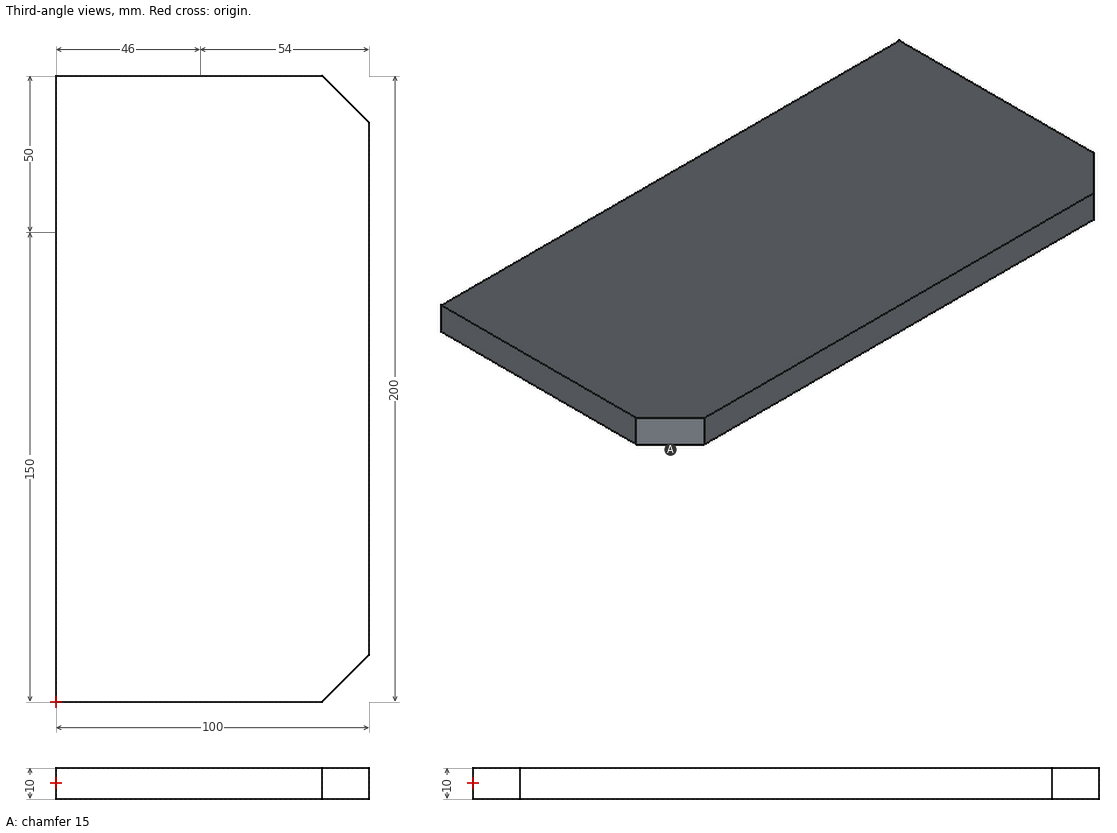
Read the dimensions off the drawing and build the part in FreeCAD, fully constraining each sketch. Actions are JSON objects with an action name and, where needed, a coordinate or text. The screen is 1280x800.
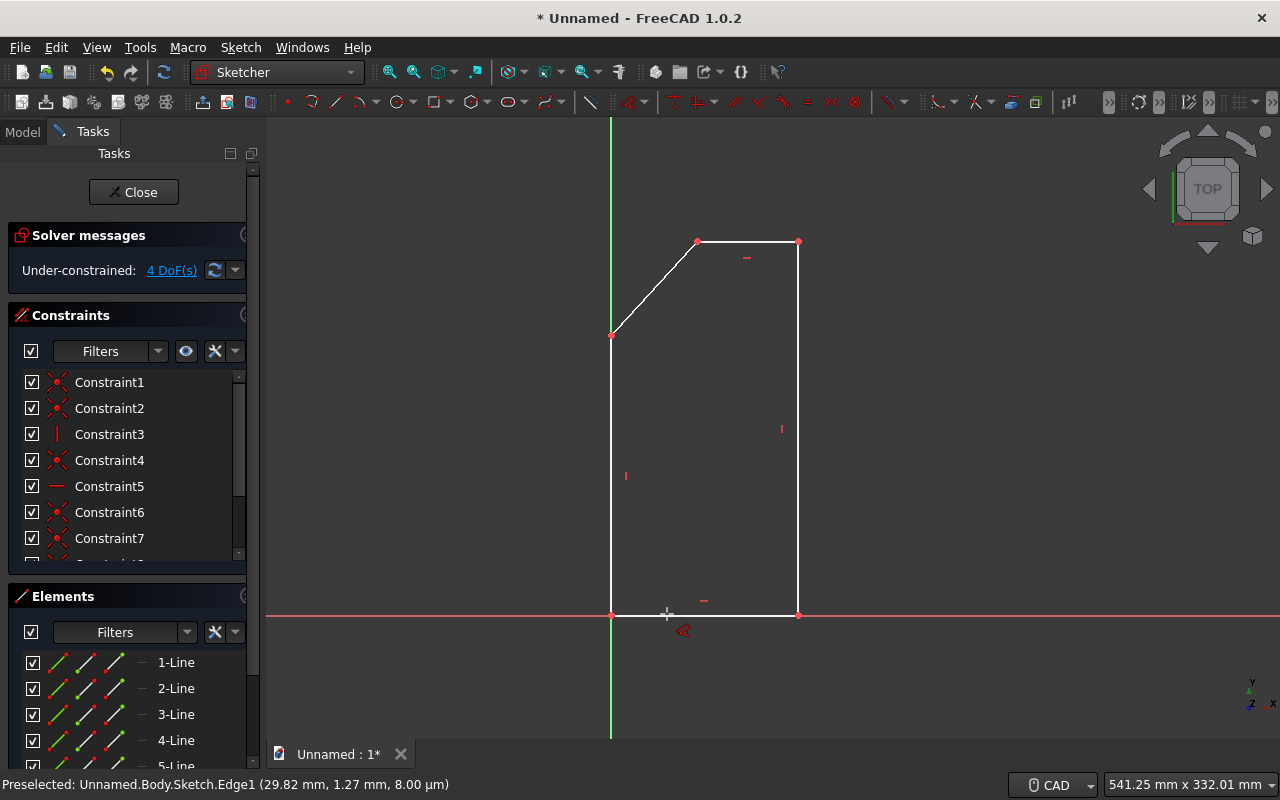
{"action": "left_click", "coordinate": [768, 242]}
{"action": "left_click", "coordinate": [747, 208]}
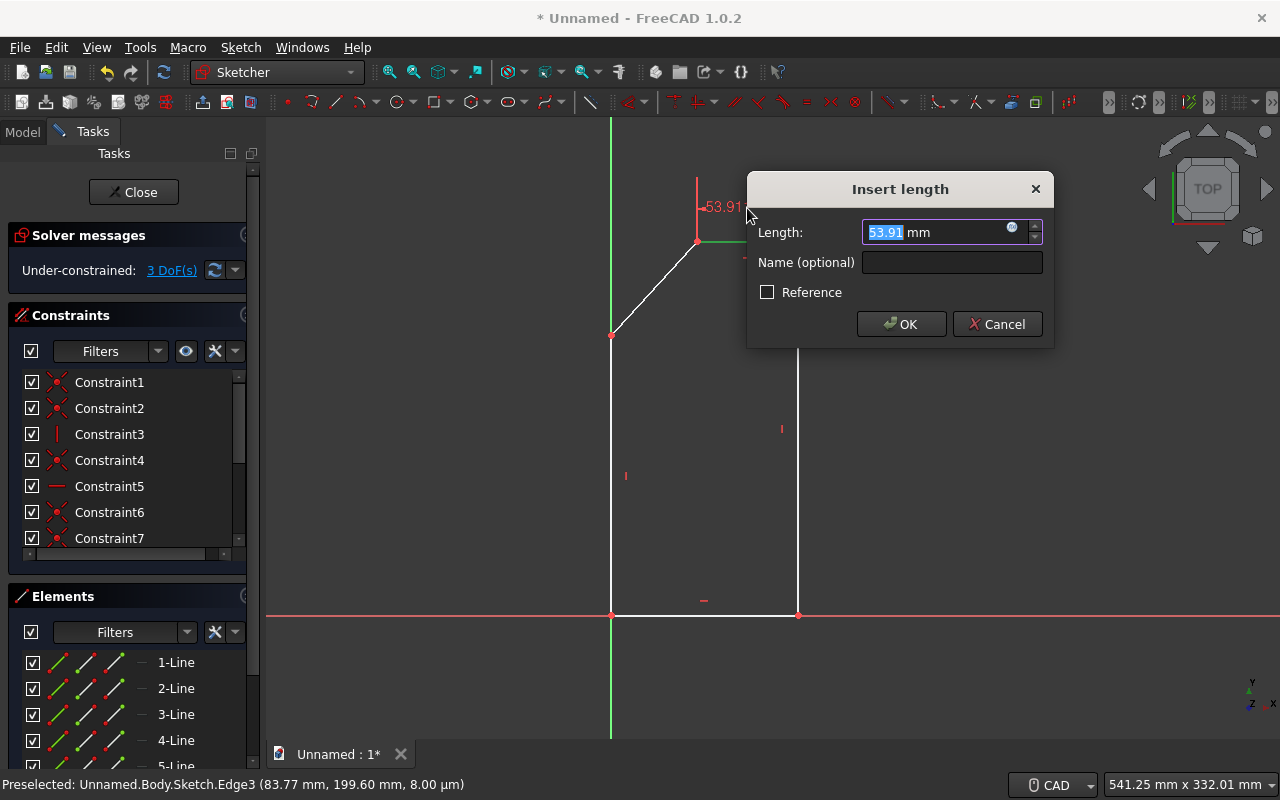
{"action": "type", "text": "54"}
{"action": "key", "text": "Return"}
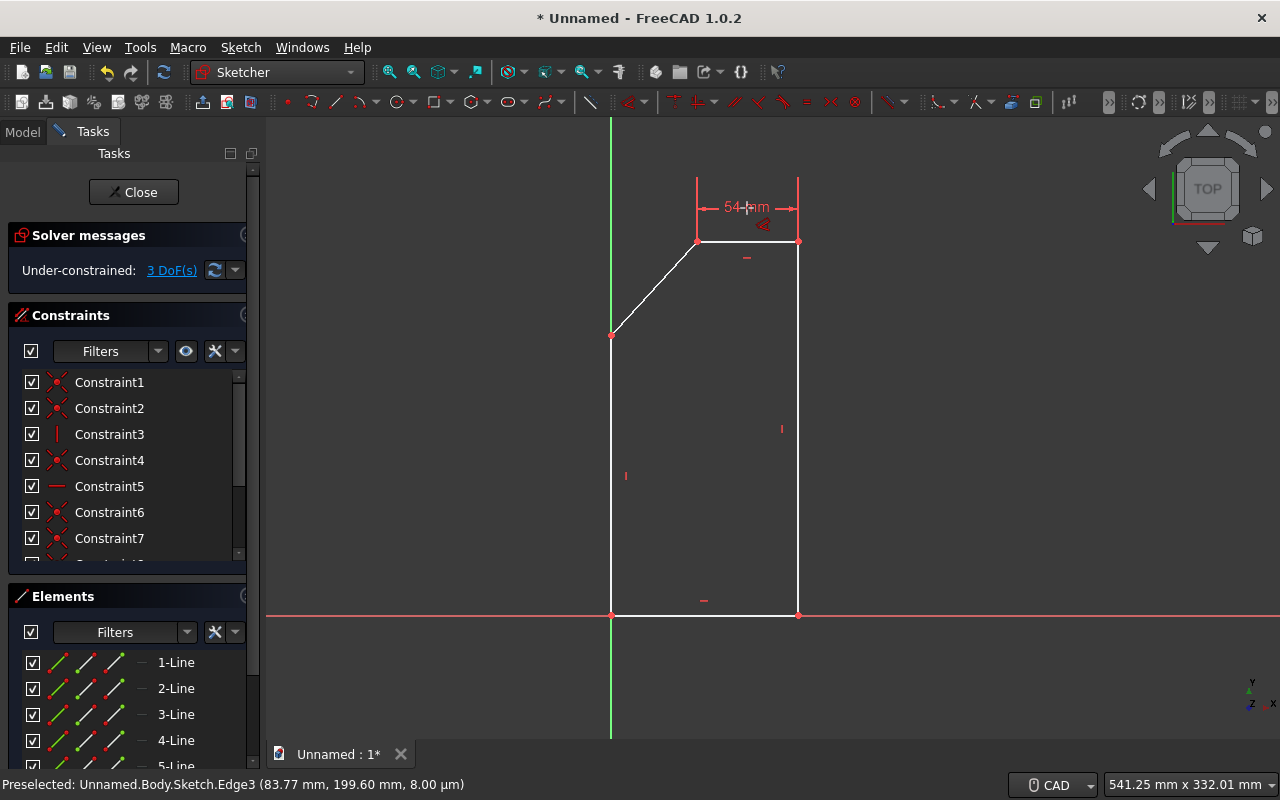
{"action": "left_click", "coordinate": [667, 616]}
{"action": "left_click", "coordinate": [705, 650]}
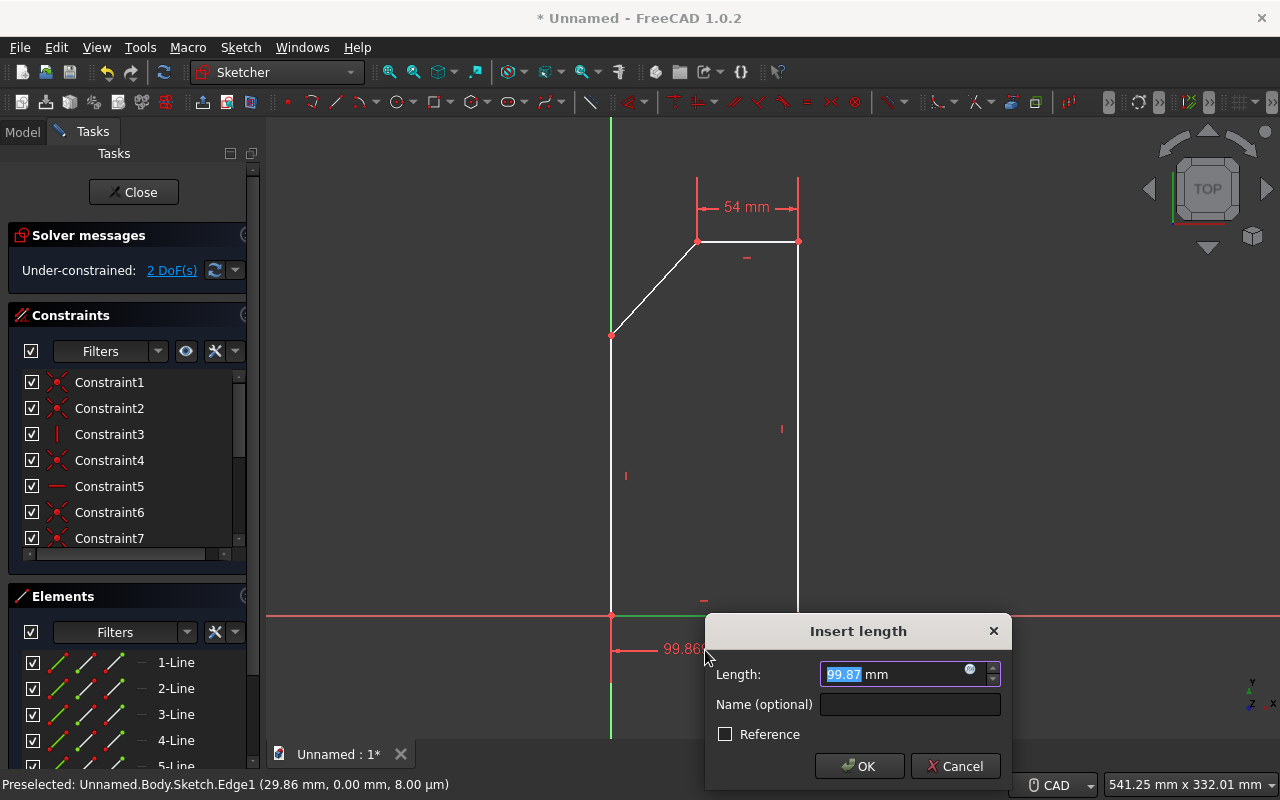
{"action": "type", "text": "100"}
{"action": "key", "text": "Return"}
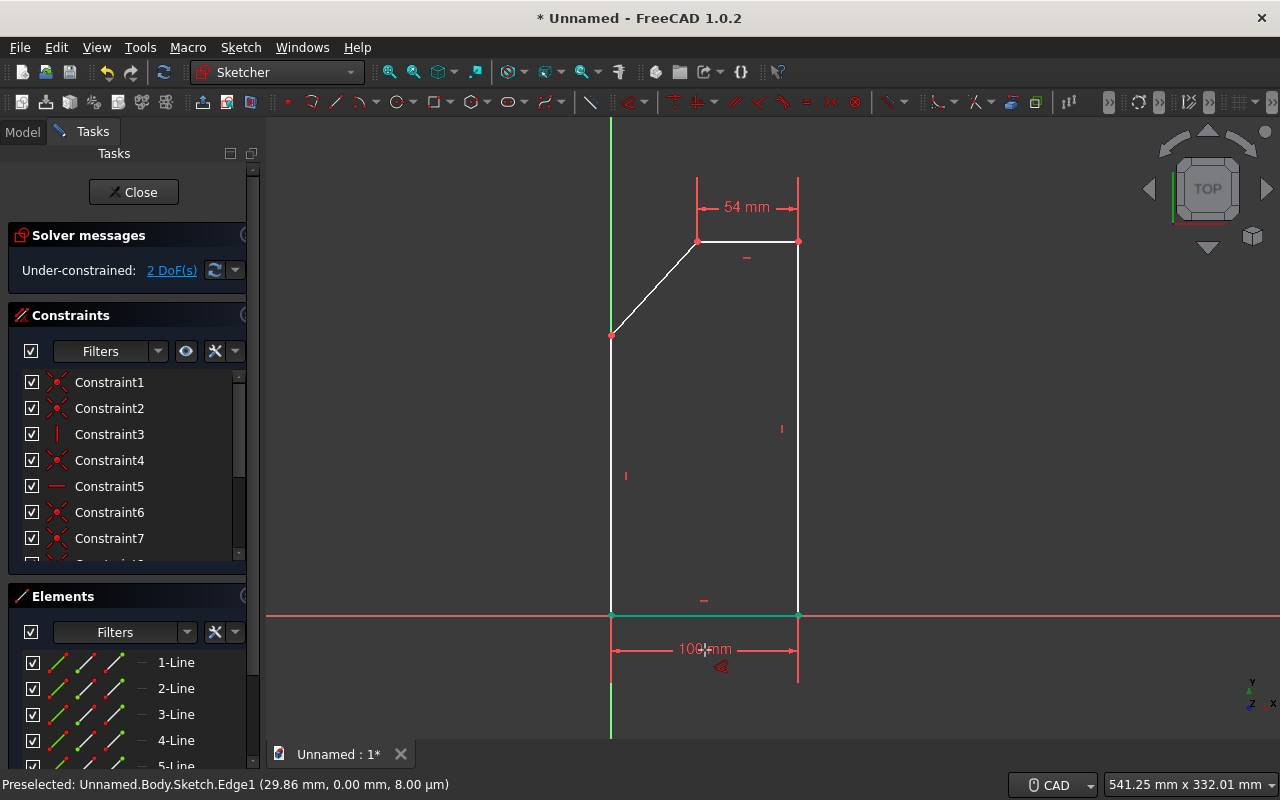
{"action": "left_click", "coordinate": [798, 504]}
{"action": "left_click", "coordinate": [832, 429]}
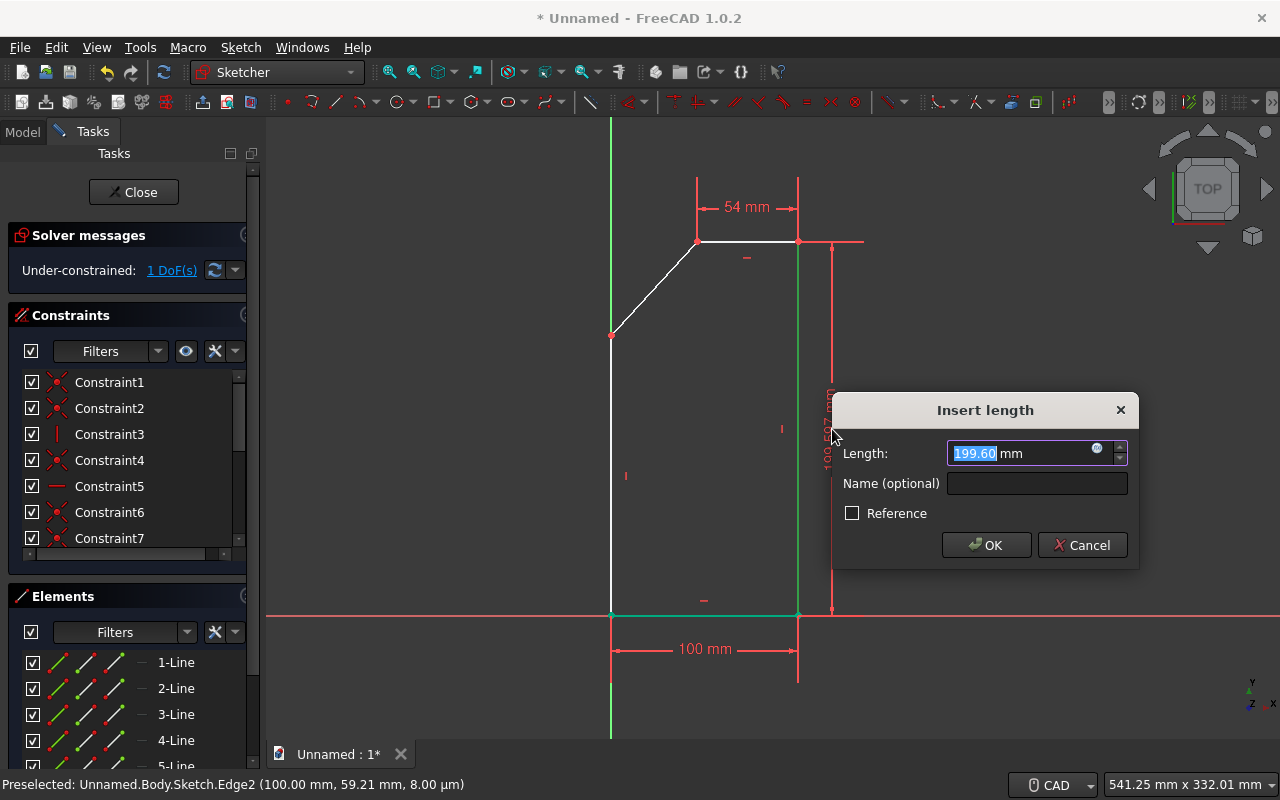
{"action": "type", "text": "200"}
{"action": "key", "text": "Return"}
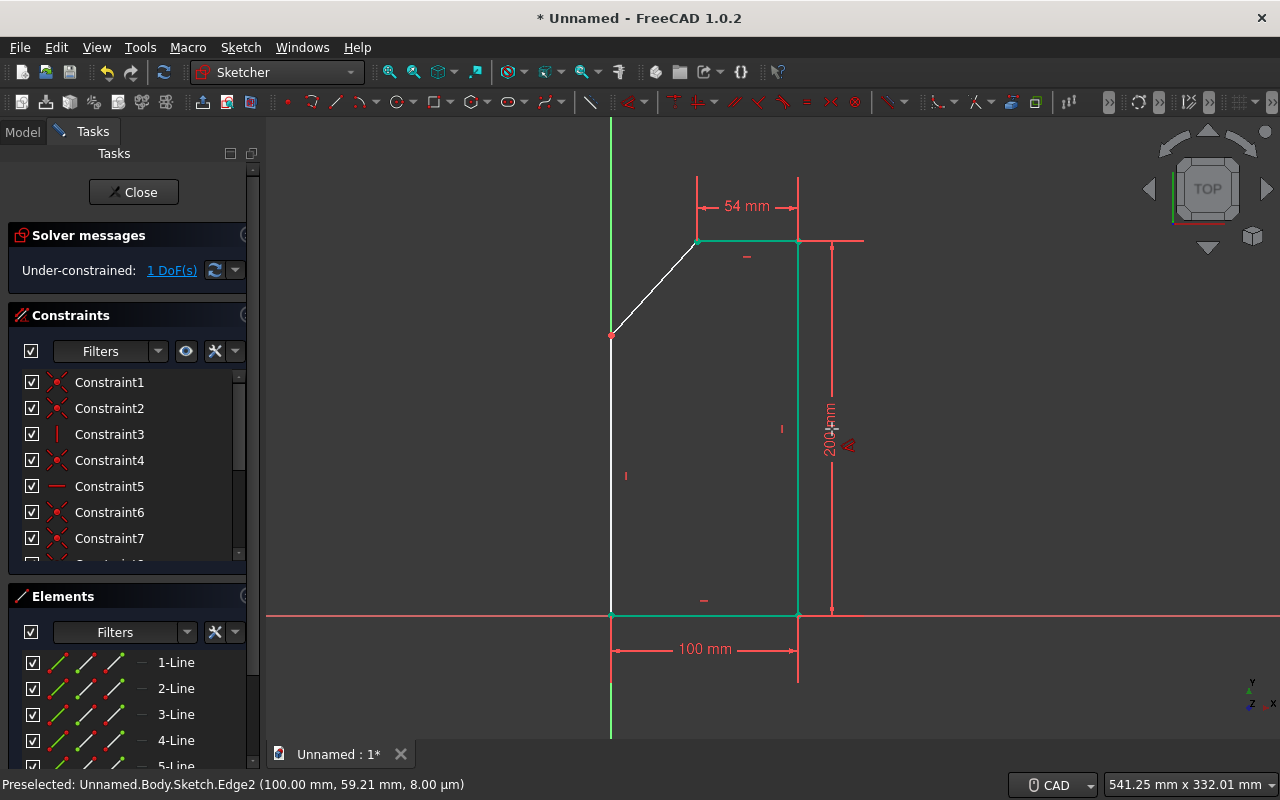
{"action": "left_click", "coordinate": [611, 420]}
{"action": "left_click", "coordinate": [577, 476]}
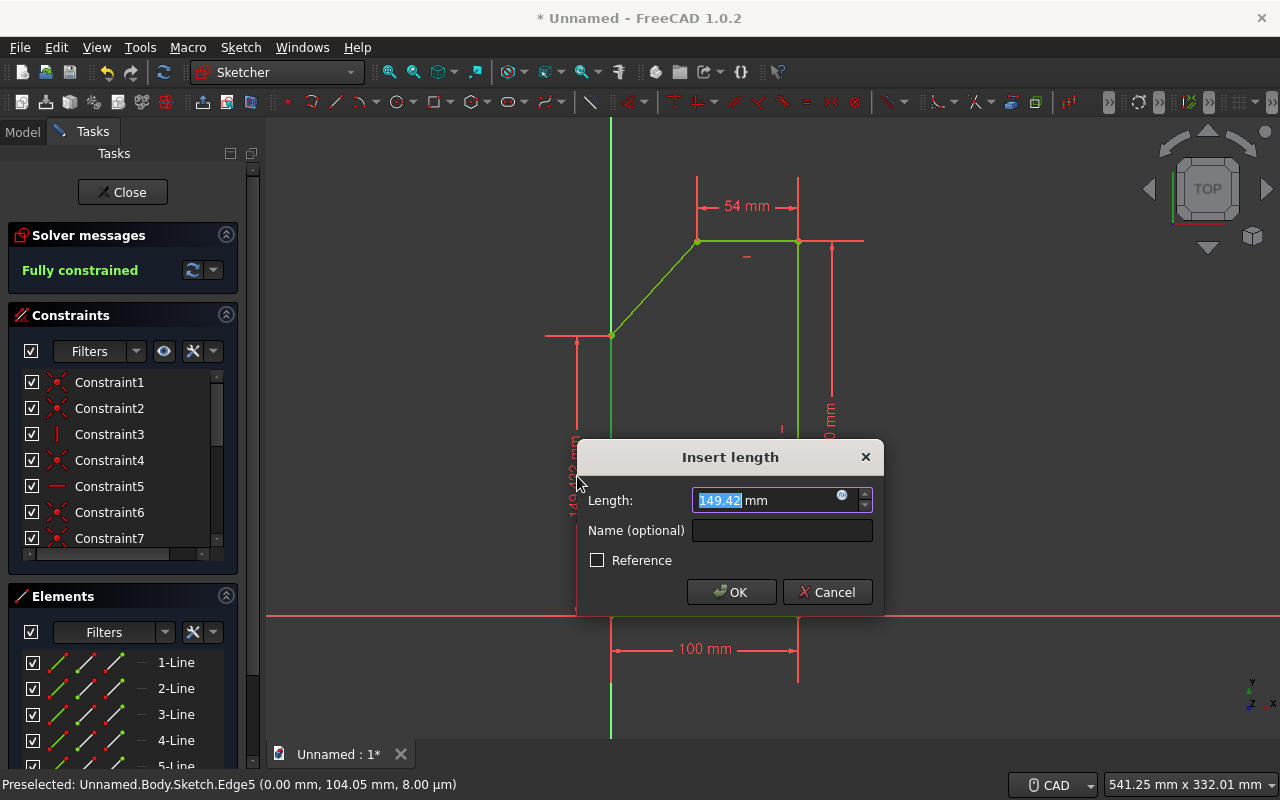
{"action": "type", "text": "150"}
{"action": "key", "text": "Return"}
{"action": "key", "text": "Escape"}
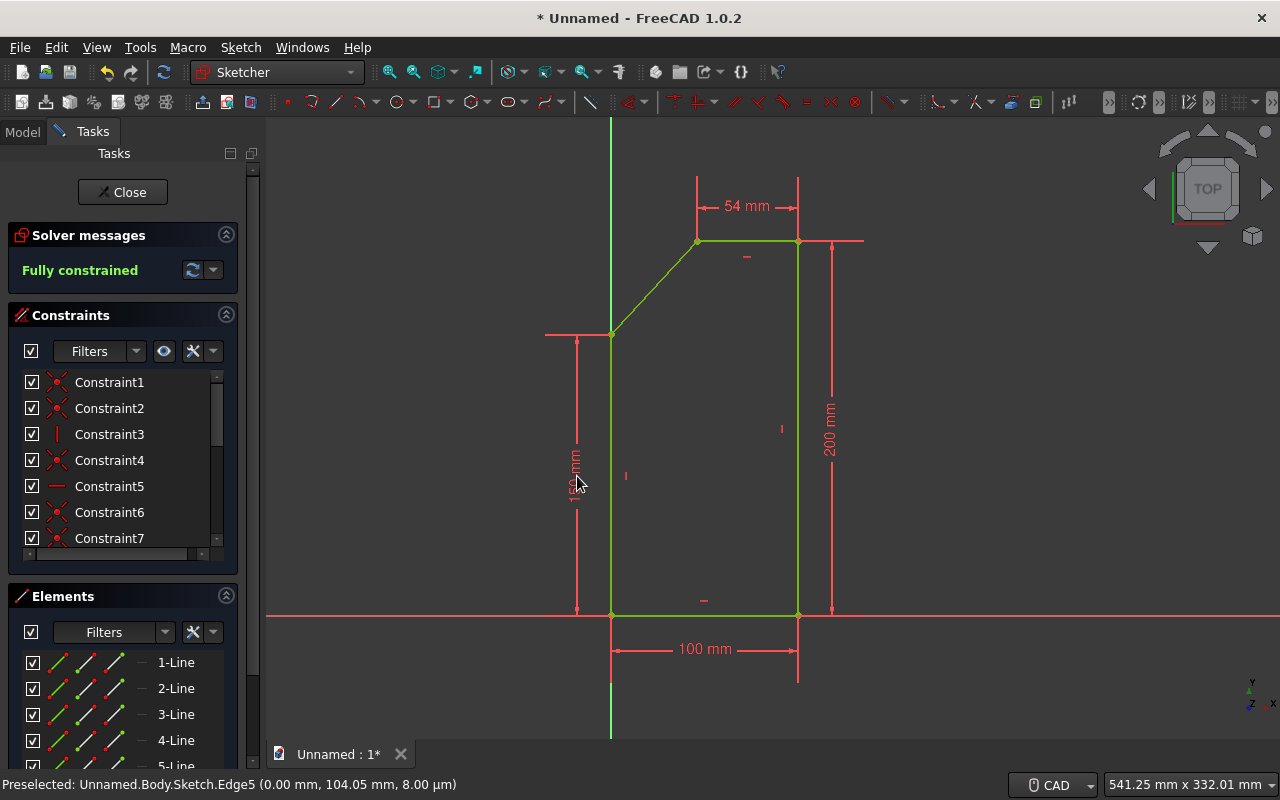
{"action": "left_click", "coordinate": [123, 192]}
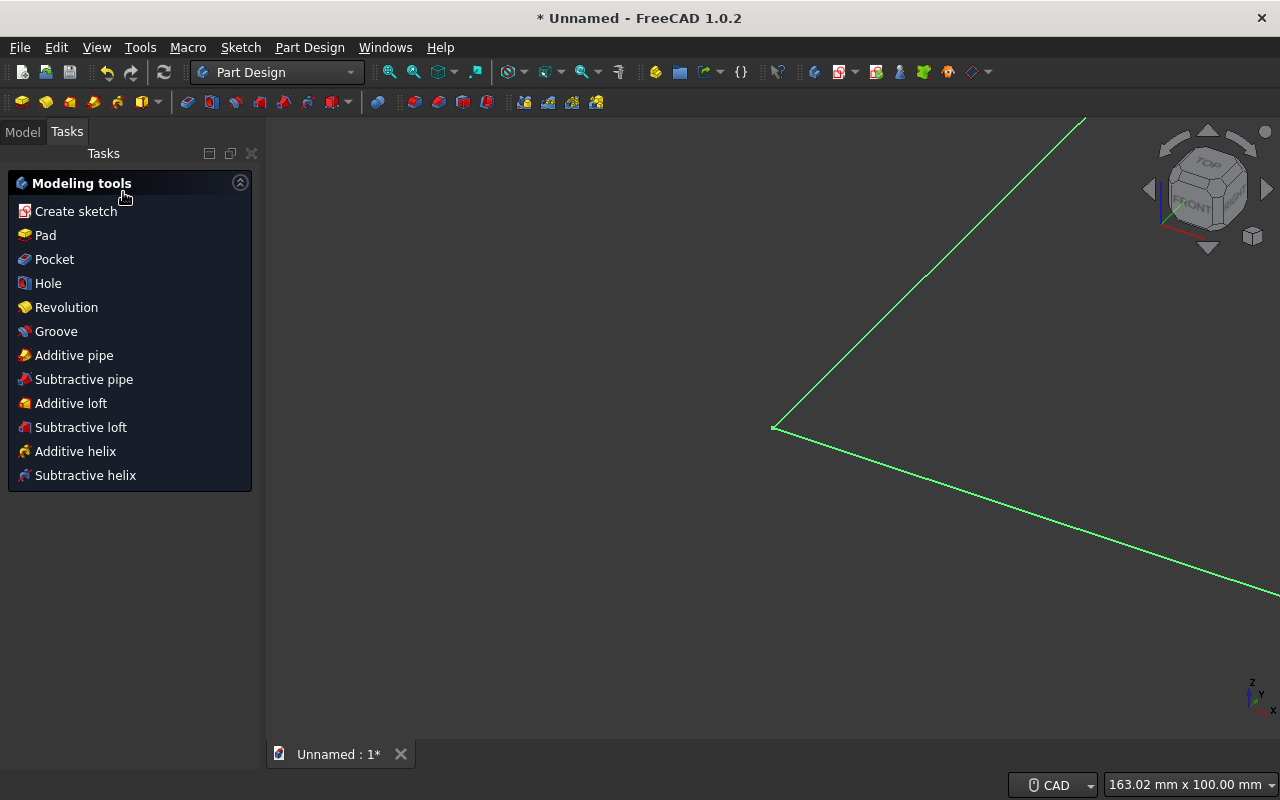
{"action": "left_click", "coordinate": [22, 102]}